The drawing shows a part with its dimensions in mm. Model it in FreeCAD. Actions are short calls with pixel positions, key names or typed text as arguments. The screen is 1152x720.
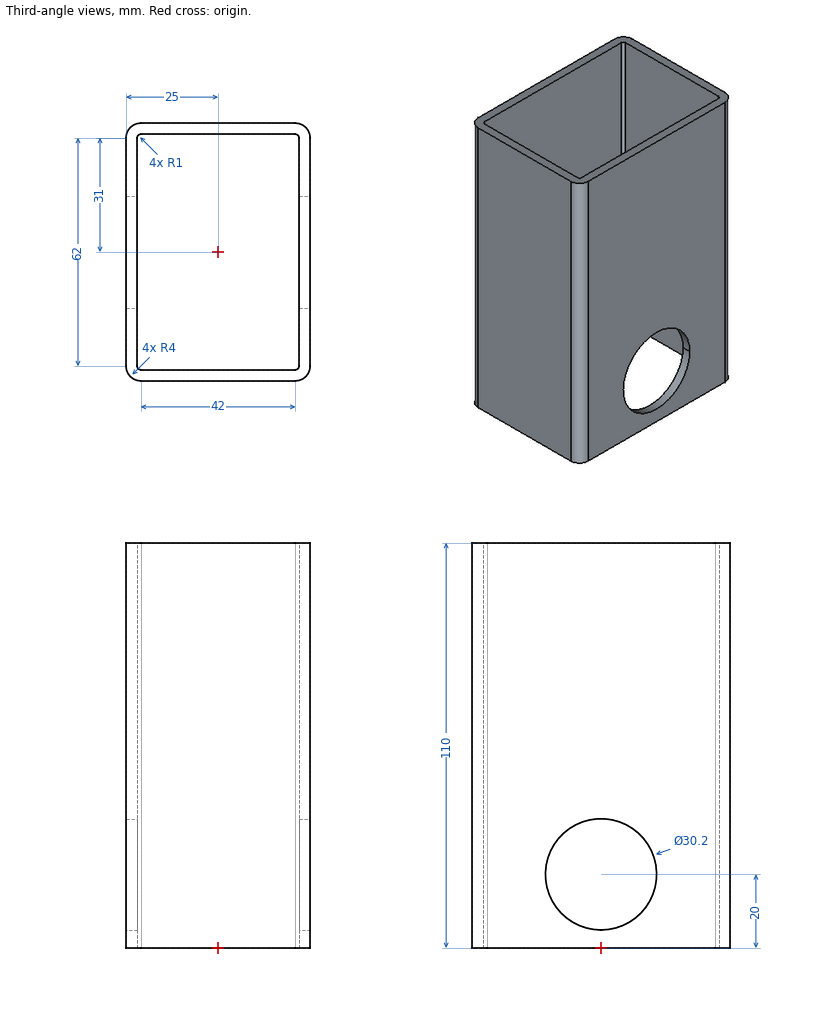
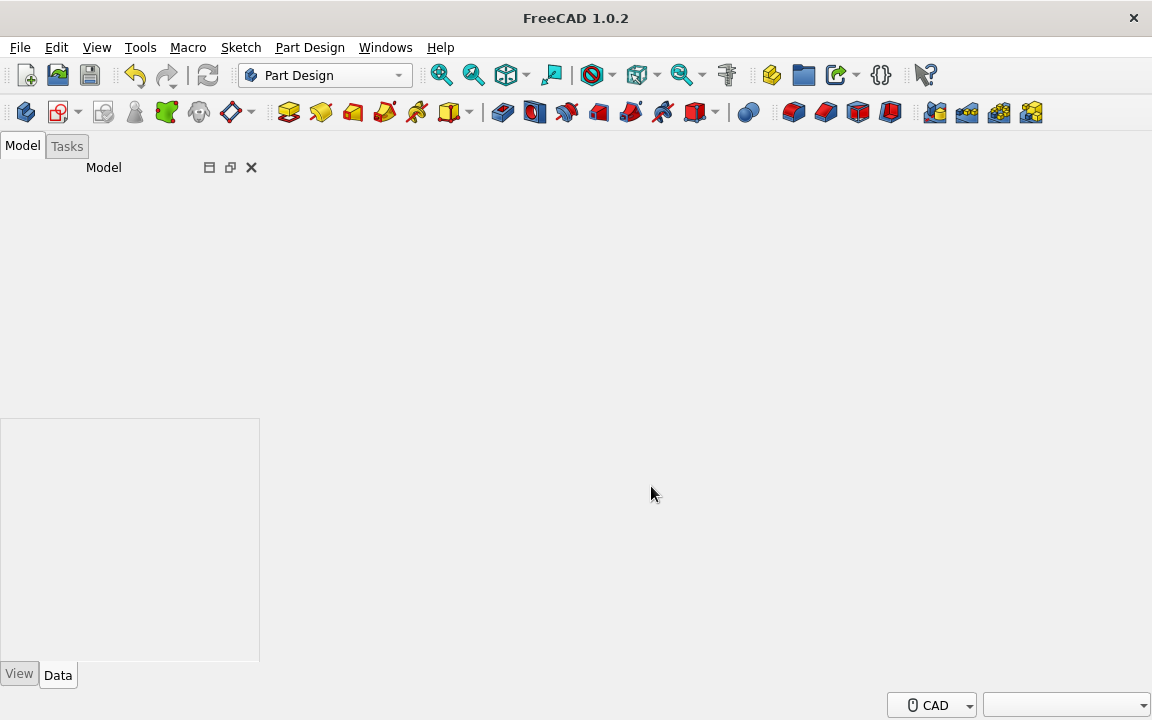
key(ctrl+n)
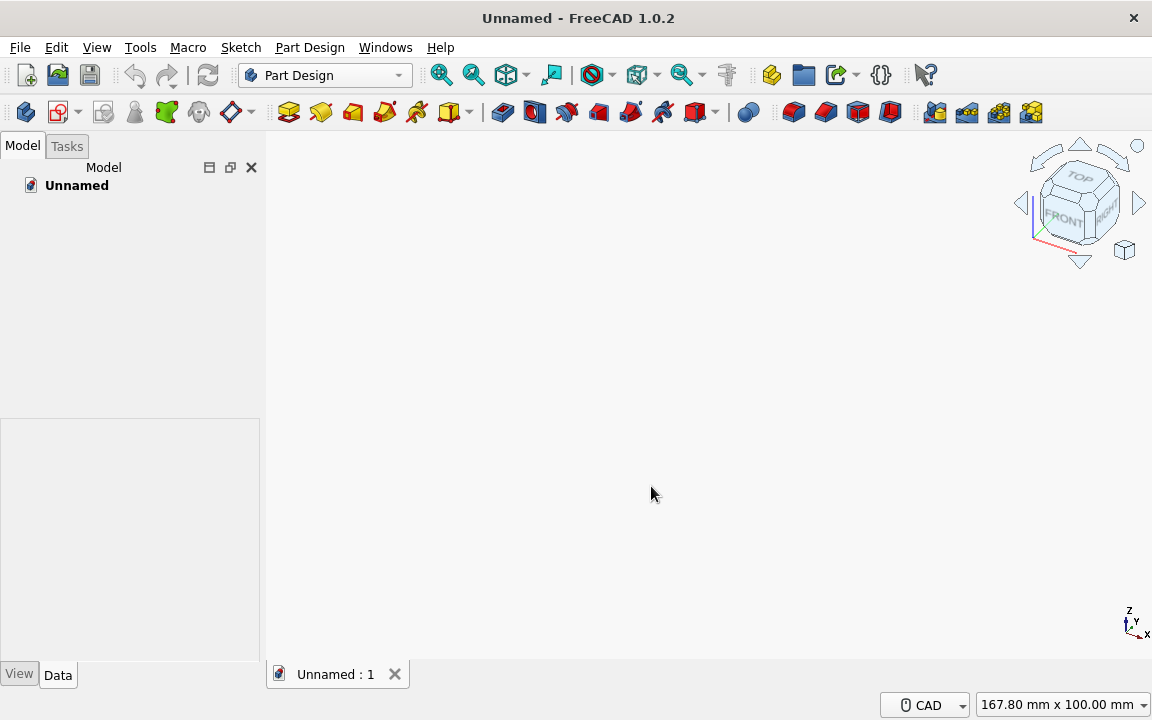
click(58, 112)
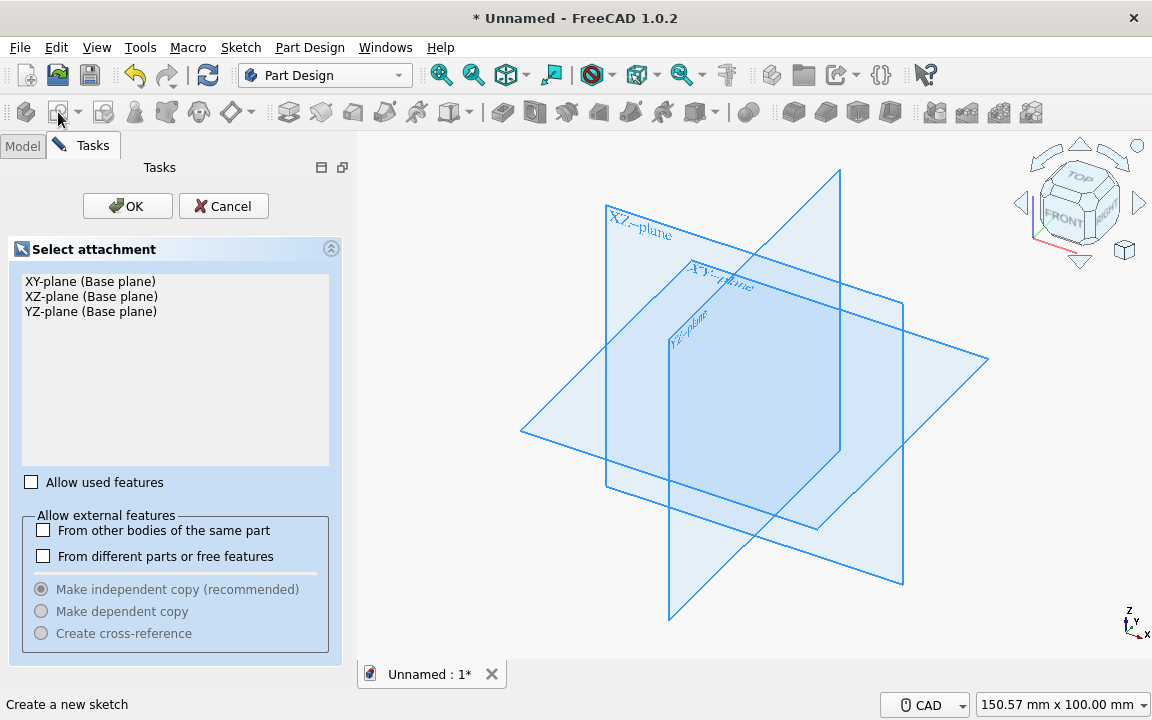
click(82, 282)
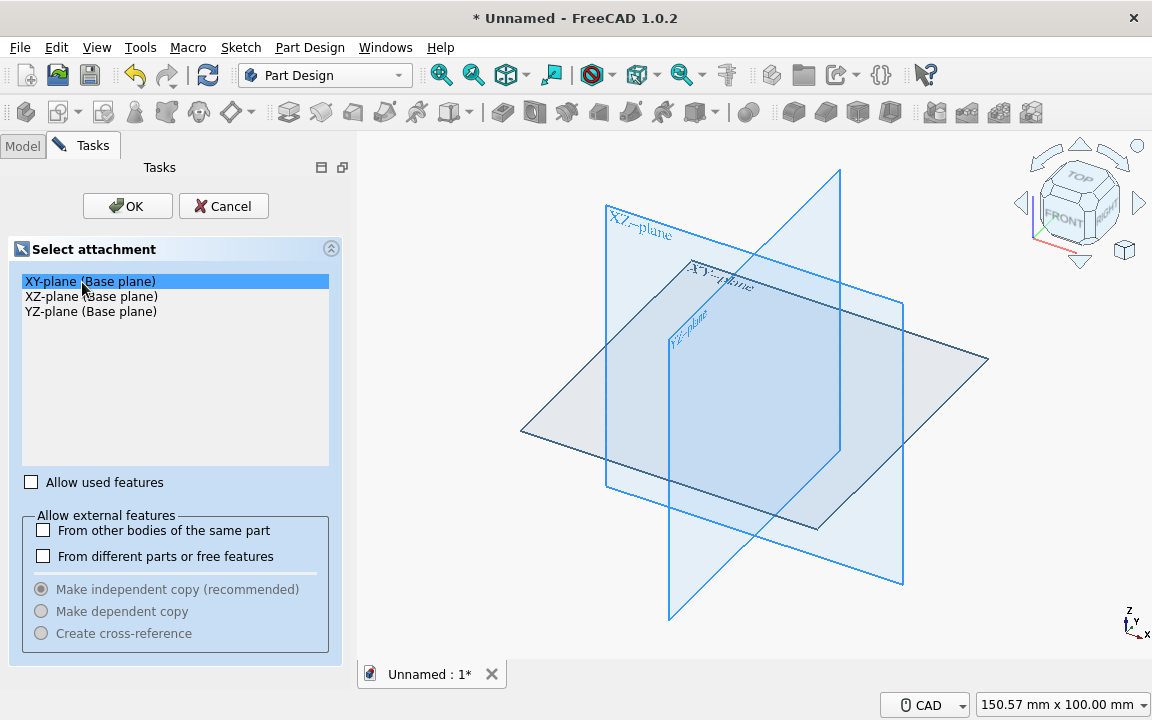
click(128, 206)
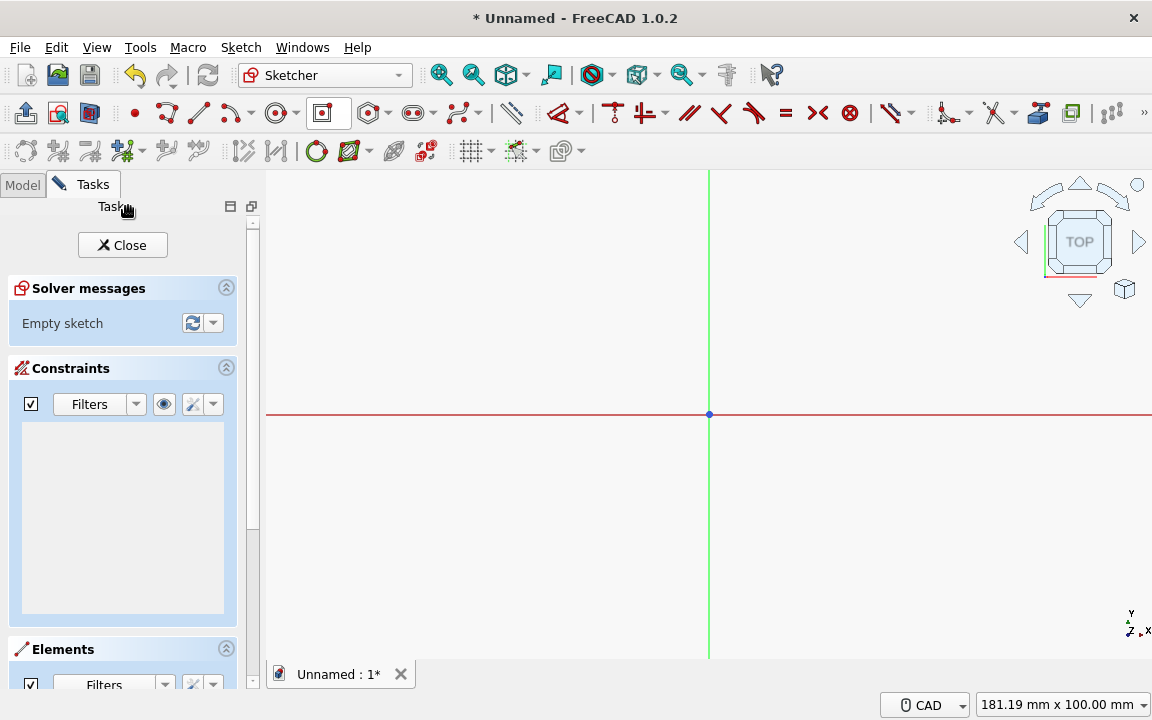
key(g)
key(l)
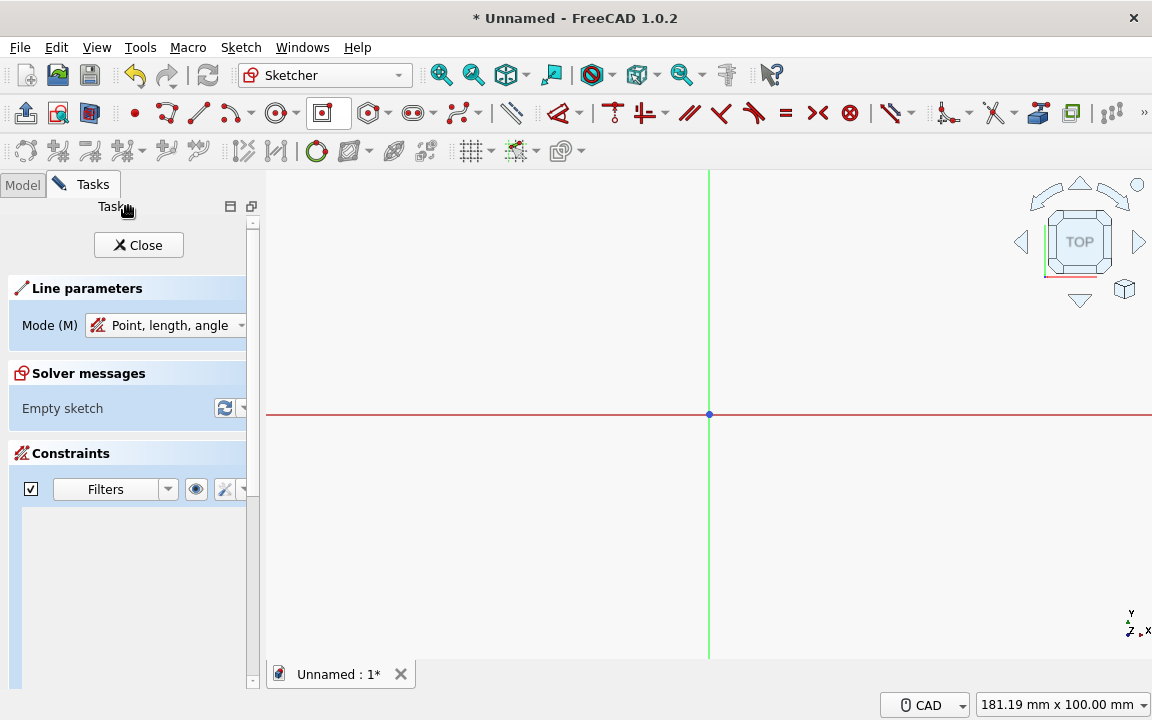
click(587, 263)
click(587, 566)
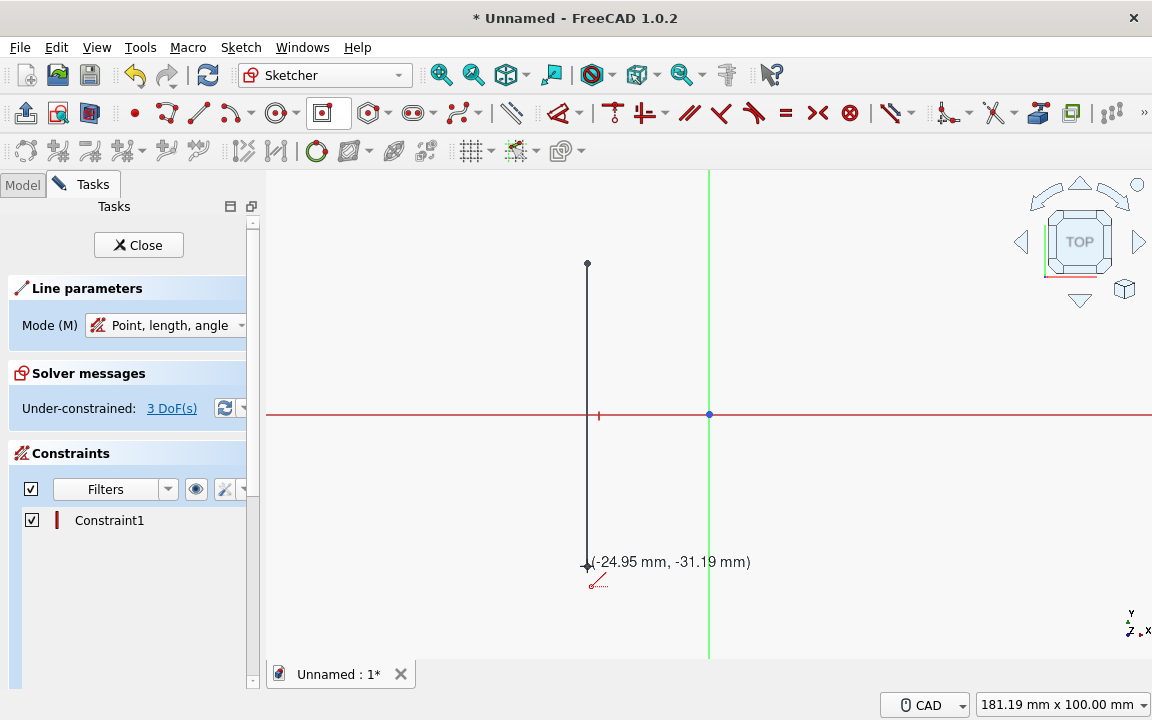
click(606, 586)
click(812, 586)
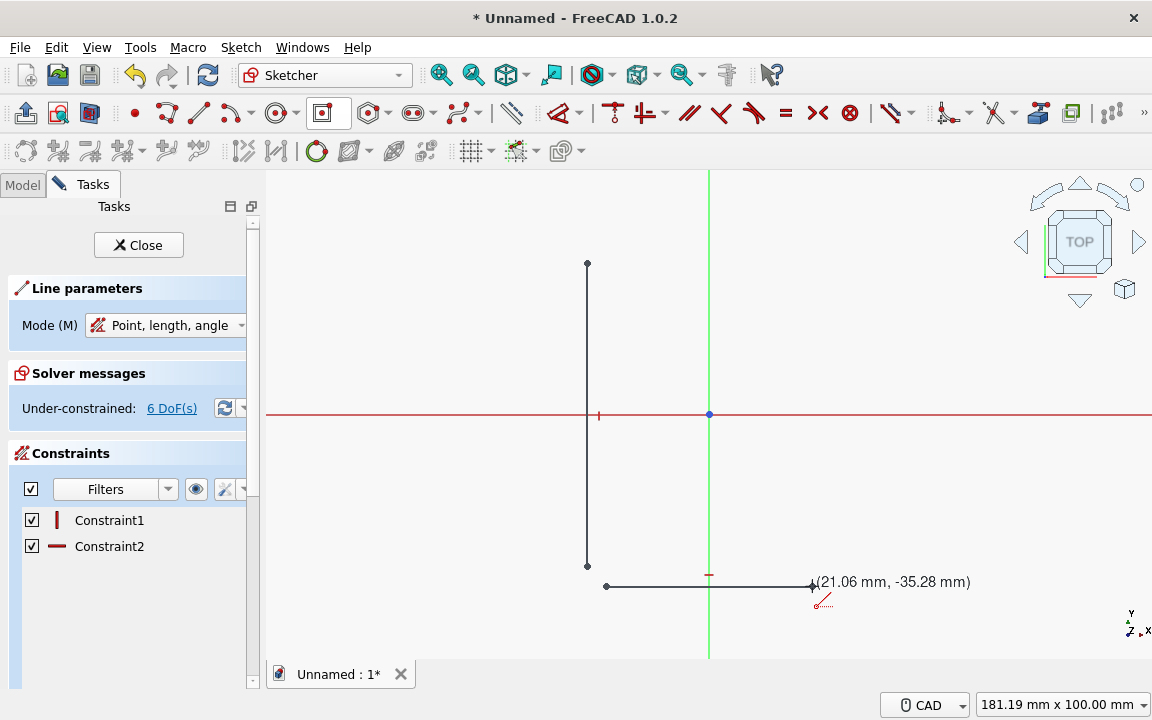
click(831, 566)
click(831, 263)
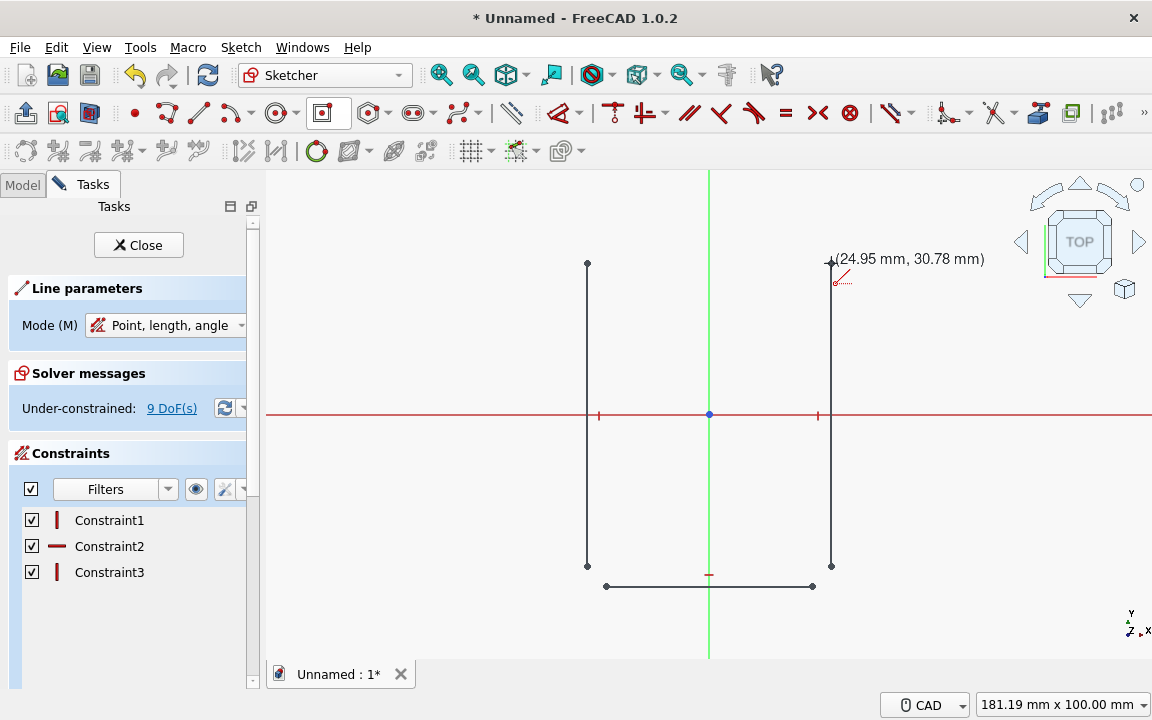
click(812, 243)
click(606, 243)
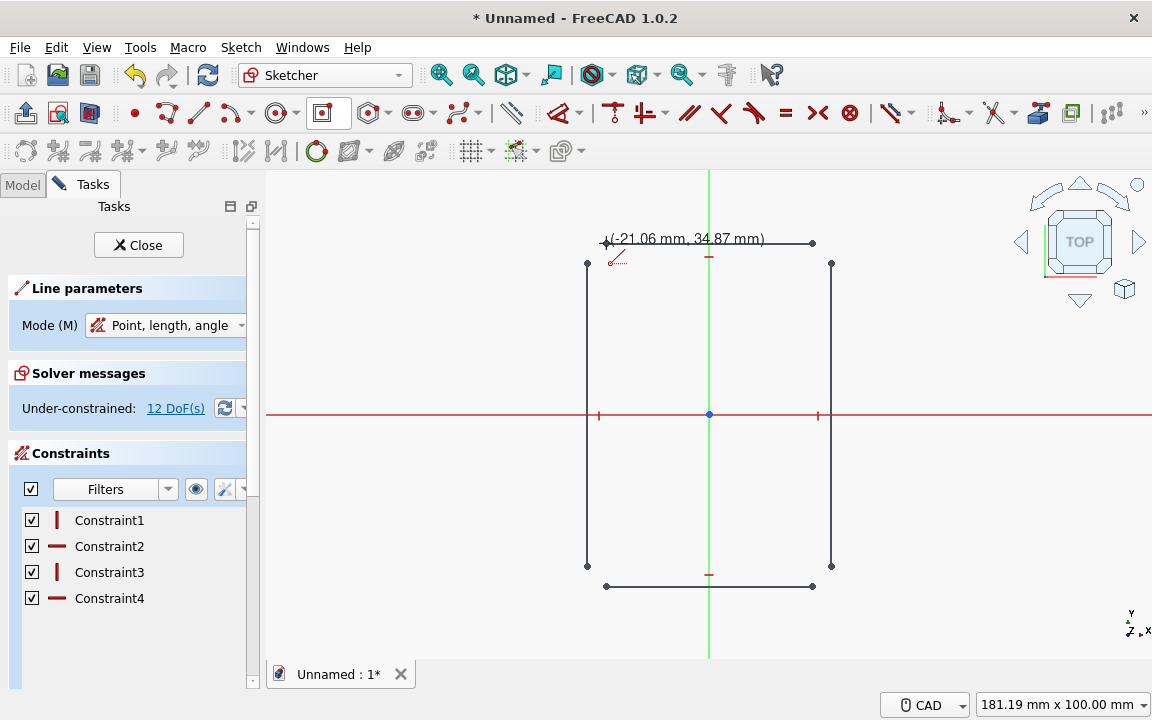
key(g)
key(3)
key(a)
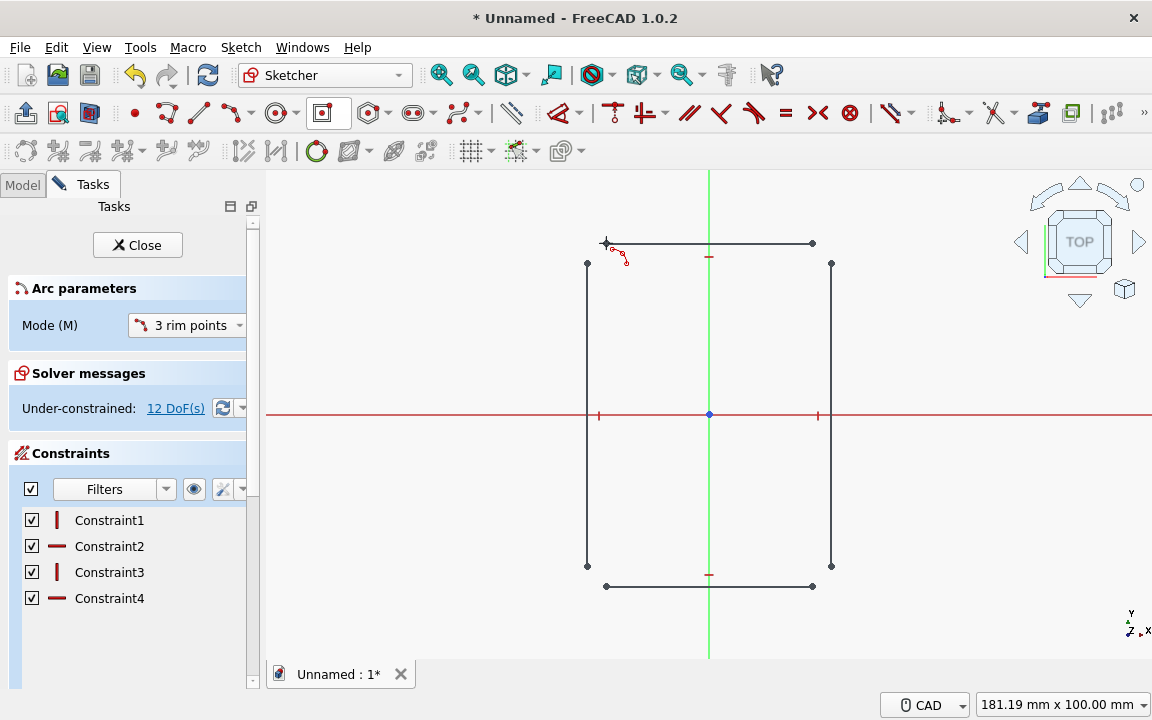
click(587, 567)
click(606, 587)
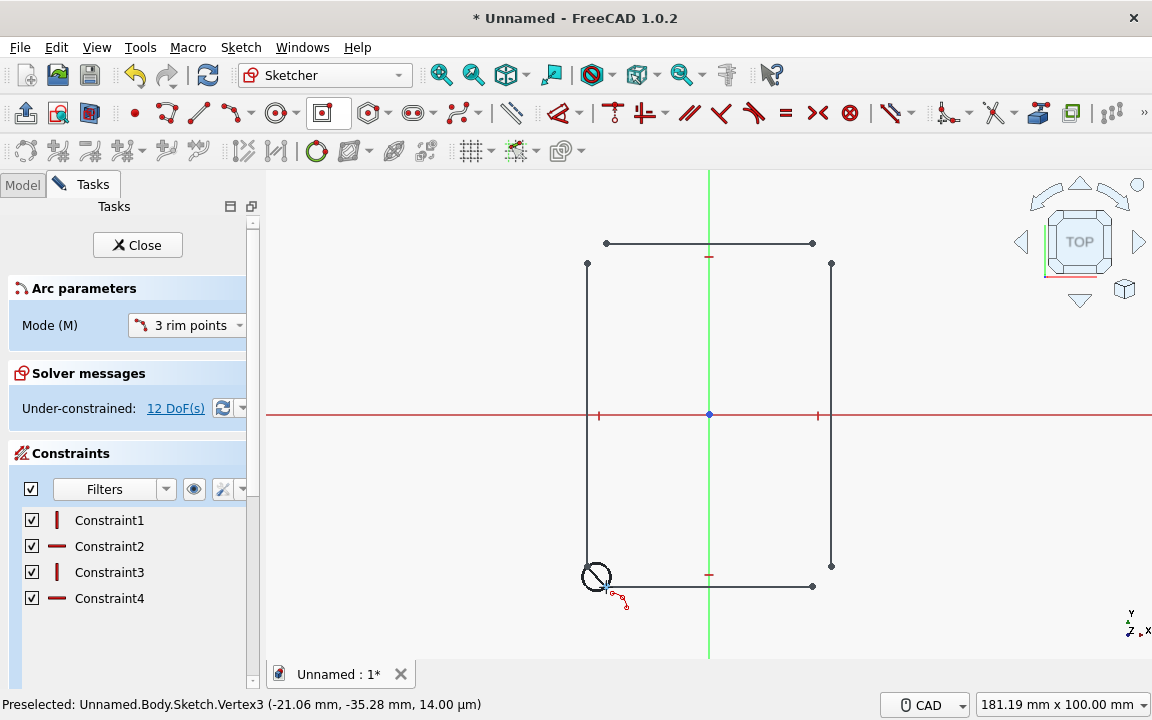
scroll(592, 580, up, 6)